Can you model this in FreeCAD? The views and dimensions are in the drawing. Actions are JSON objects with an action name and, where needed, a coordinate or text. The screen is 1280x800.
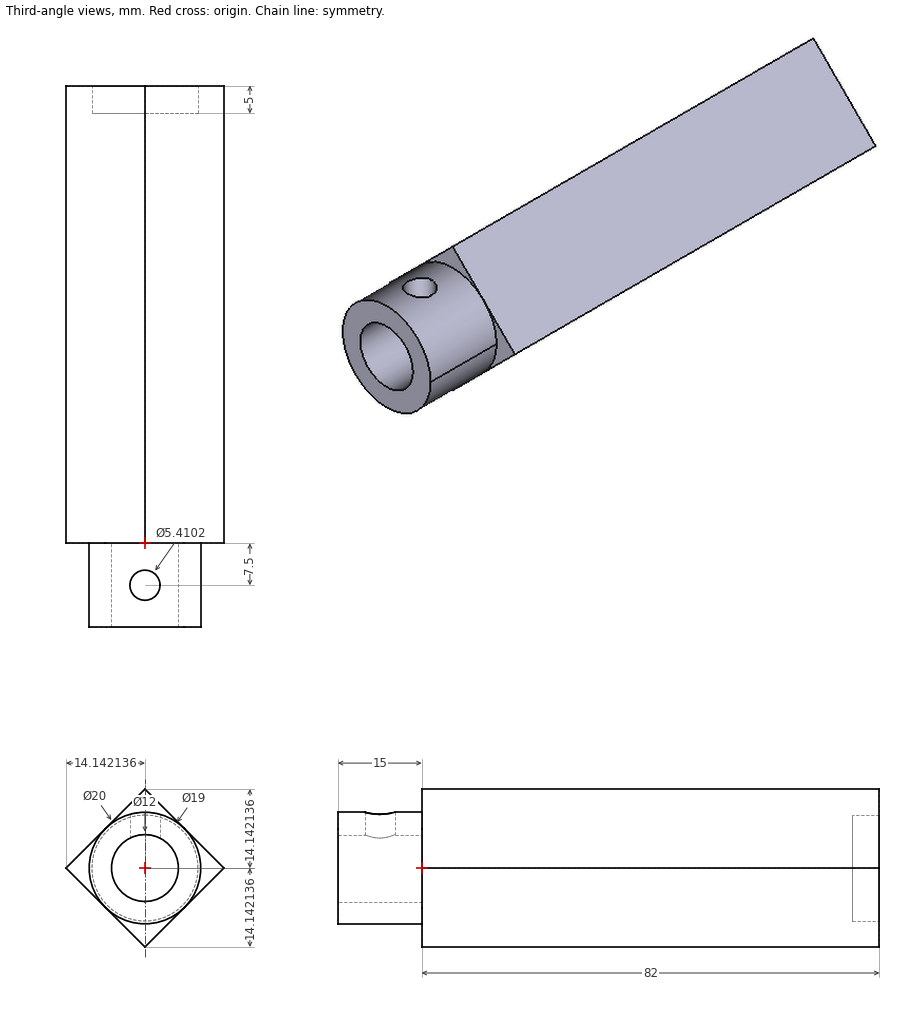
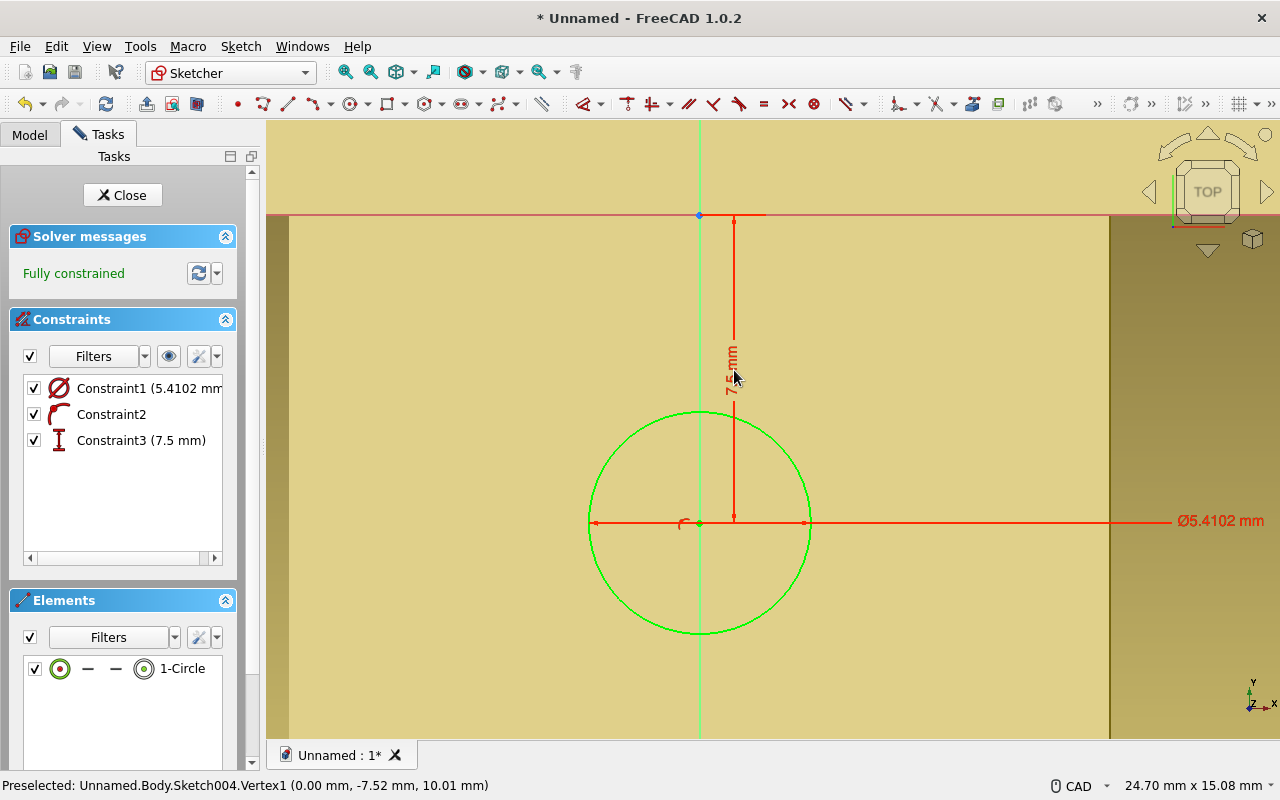
{"action": "left_click", "coordinate": [123, 195]}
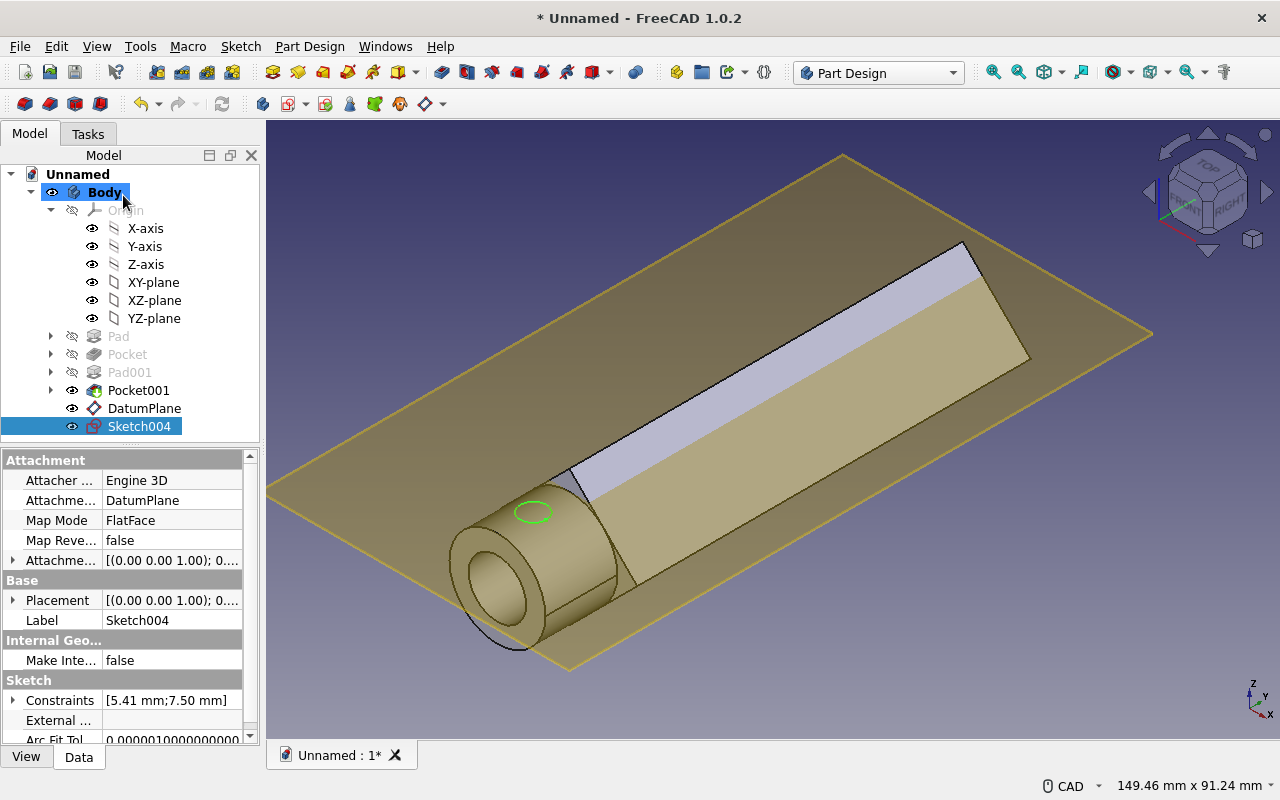
{"action": "left_click", "coordinate": [442, 72]}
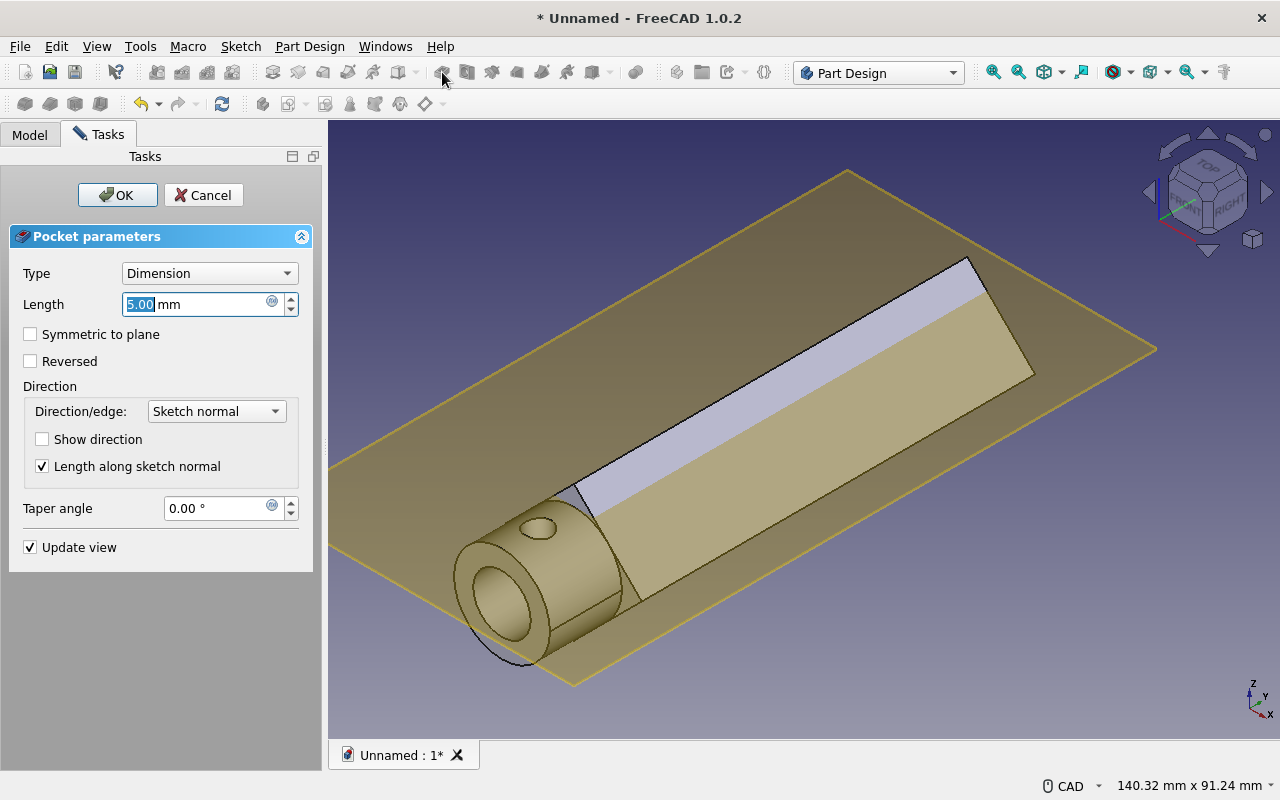
{"action": "left_click", "coordinate": [210, 274]}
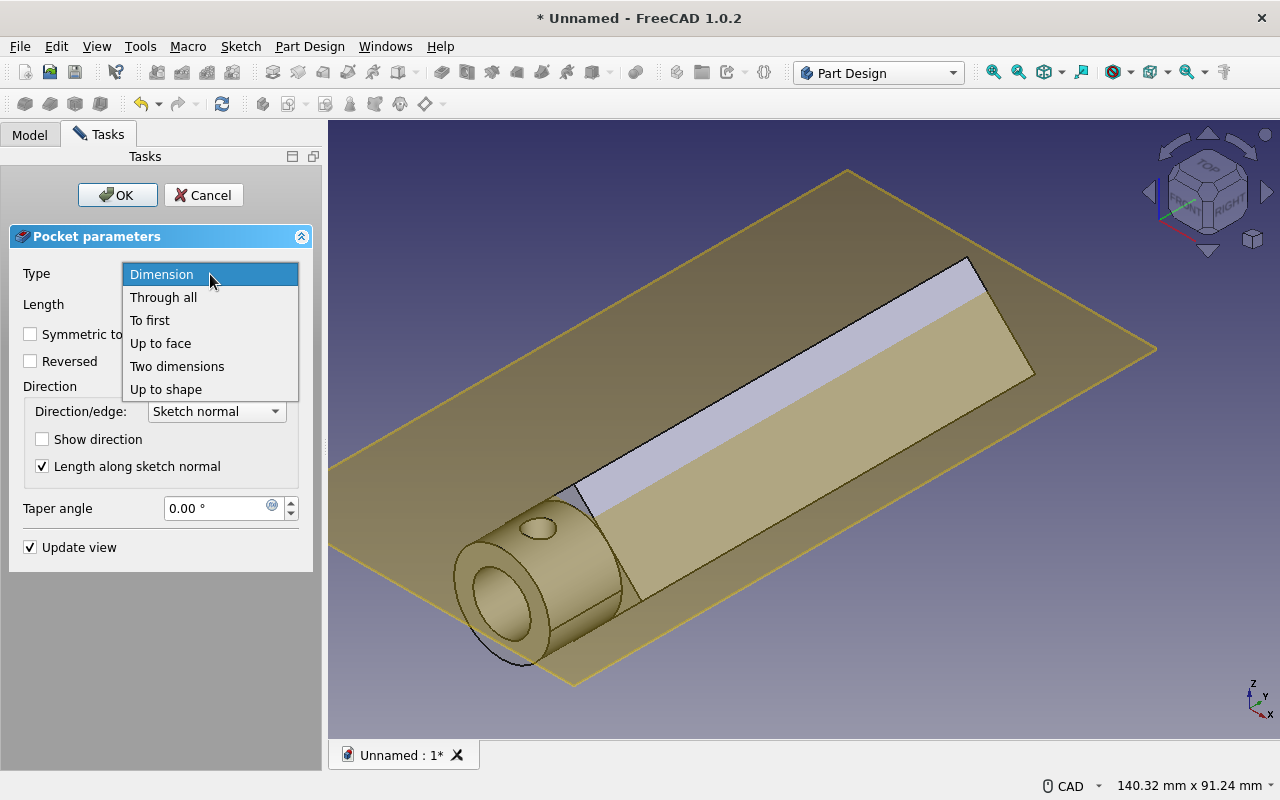
{"action": "left_click", "coordinate": [208, 320]}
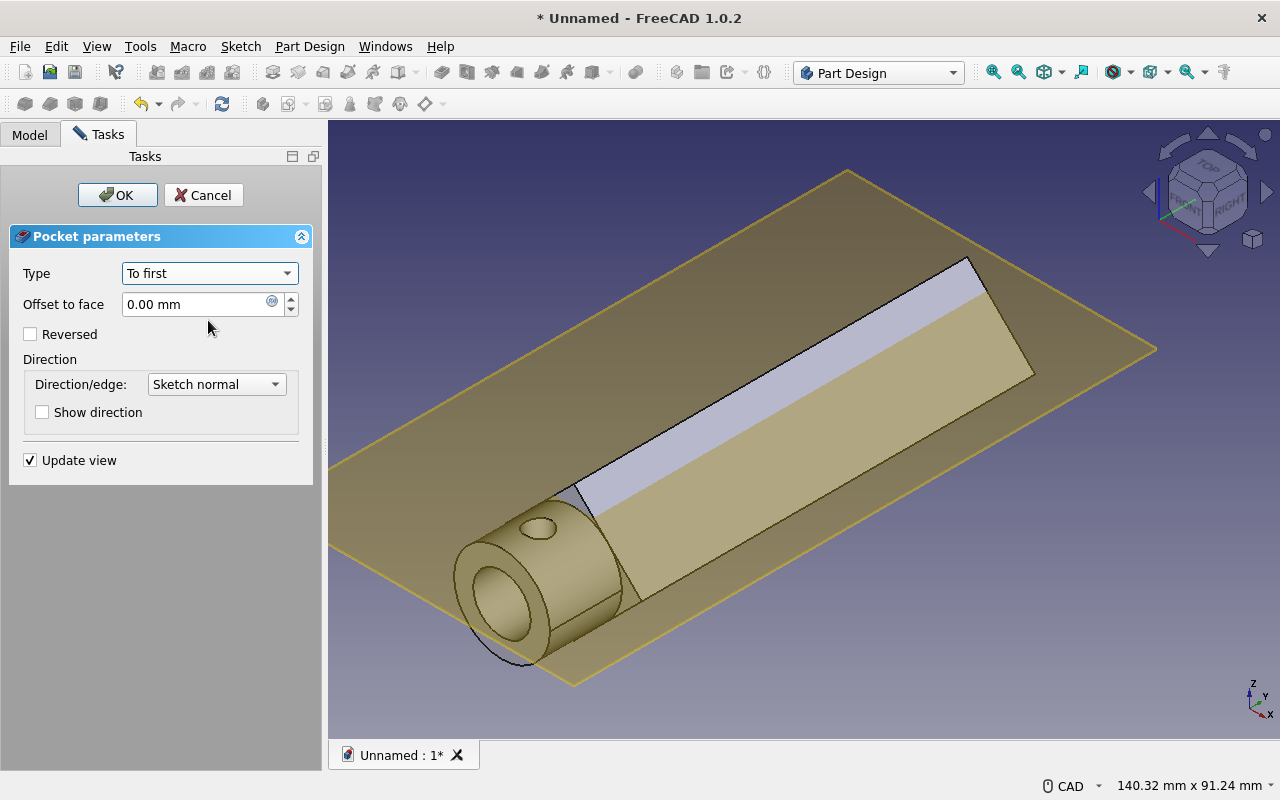
{"action": "left_click", "coordinate": [118, 195]}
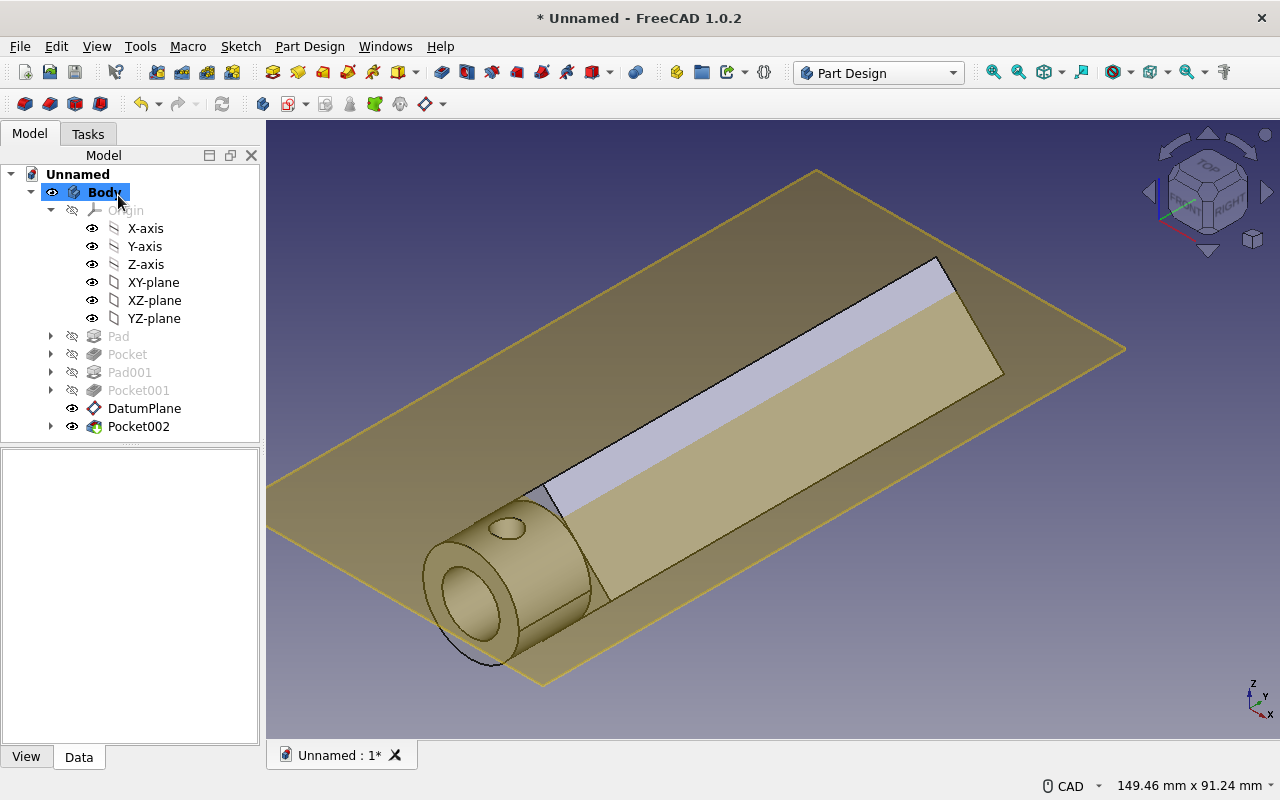
{"action": "left_click", "coordinate": [117, 408]}
{"action": "key", "text": "space"}